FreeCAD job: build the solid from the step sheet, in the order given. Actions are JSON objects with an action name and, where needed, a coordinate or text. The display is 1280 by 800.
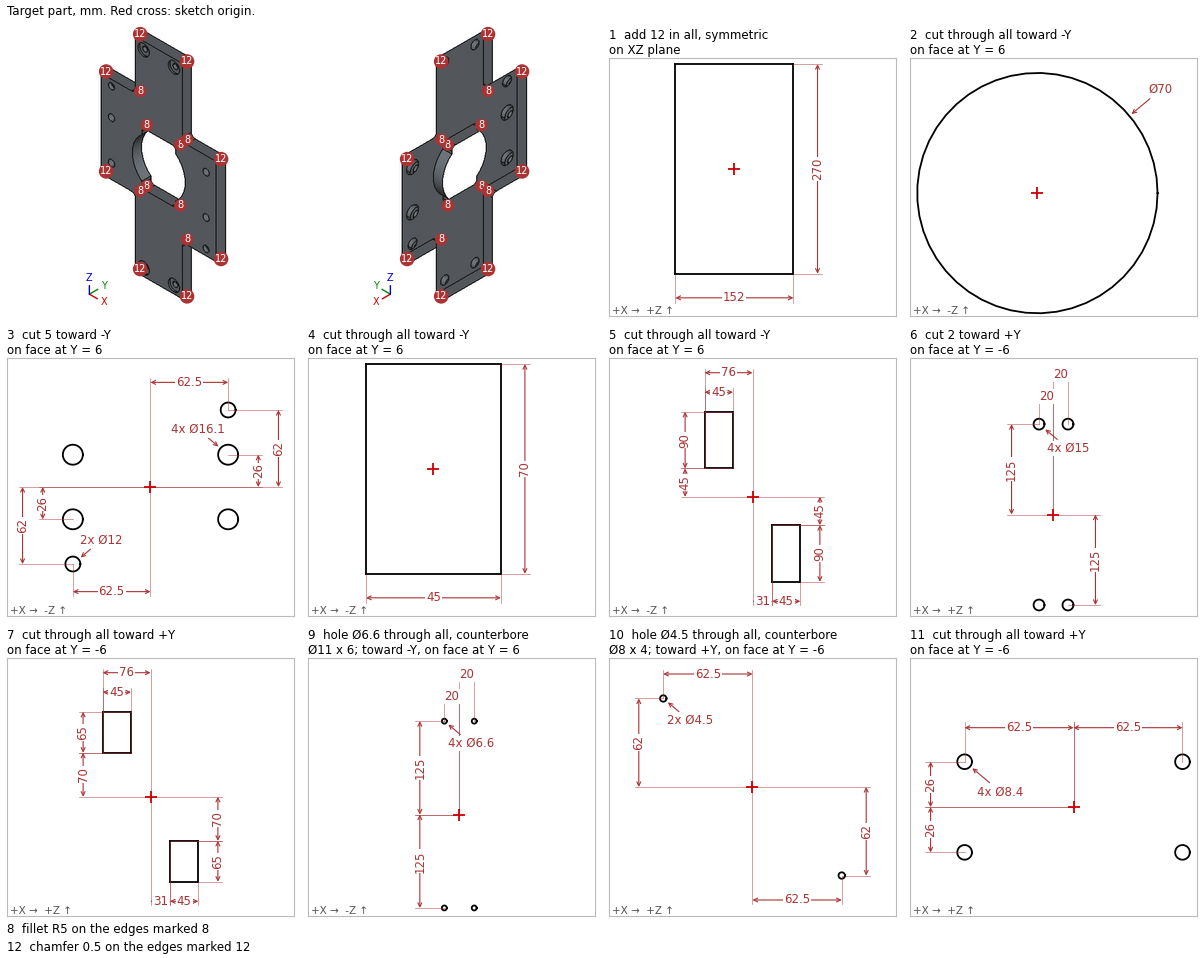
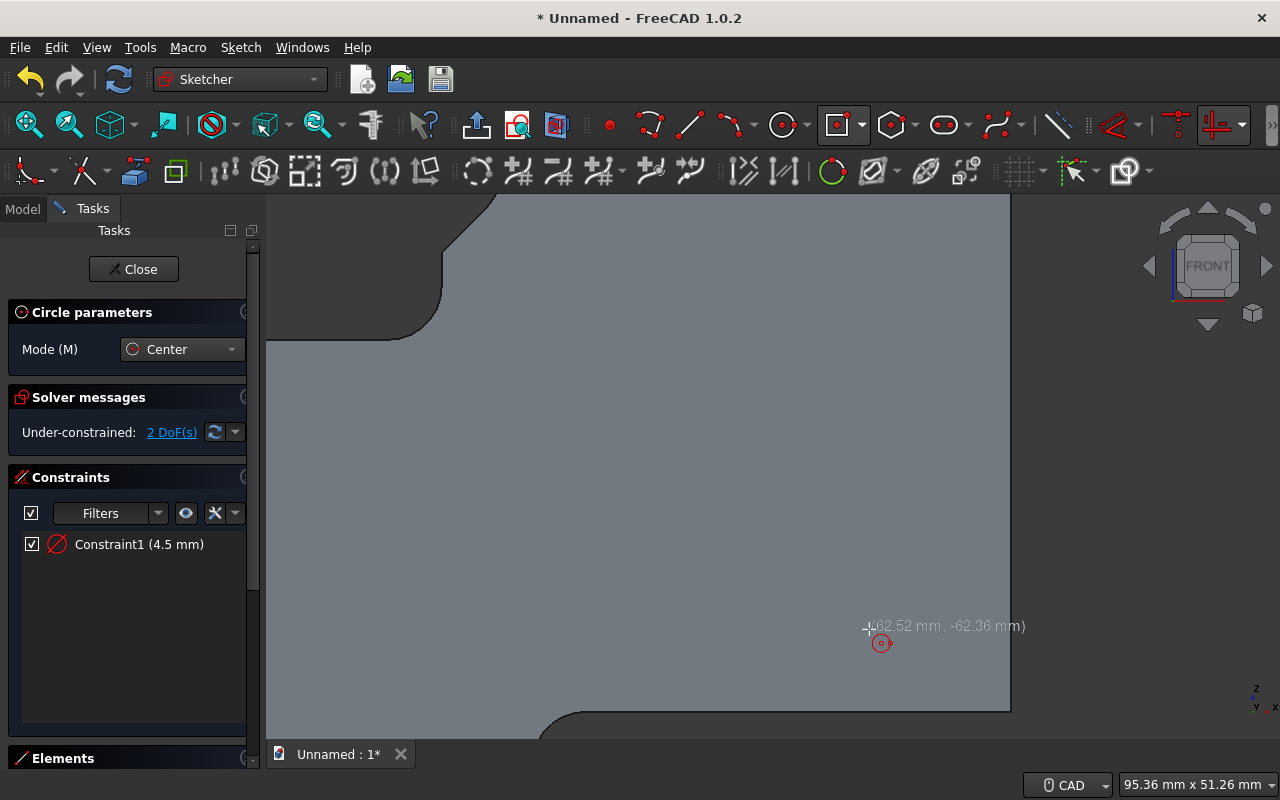
{"action": "scroll", "coordinate": [869, 630], "scroll_direction": "down", "scroll_amount": 7}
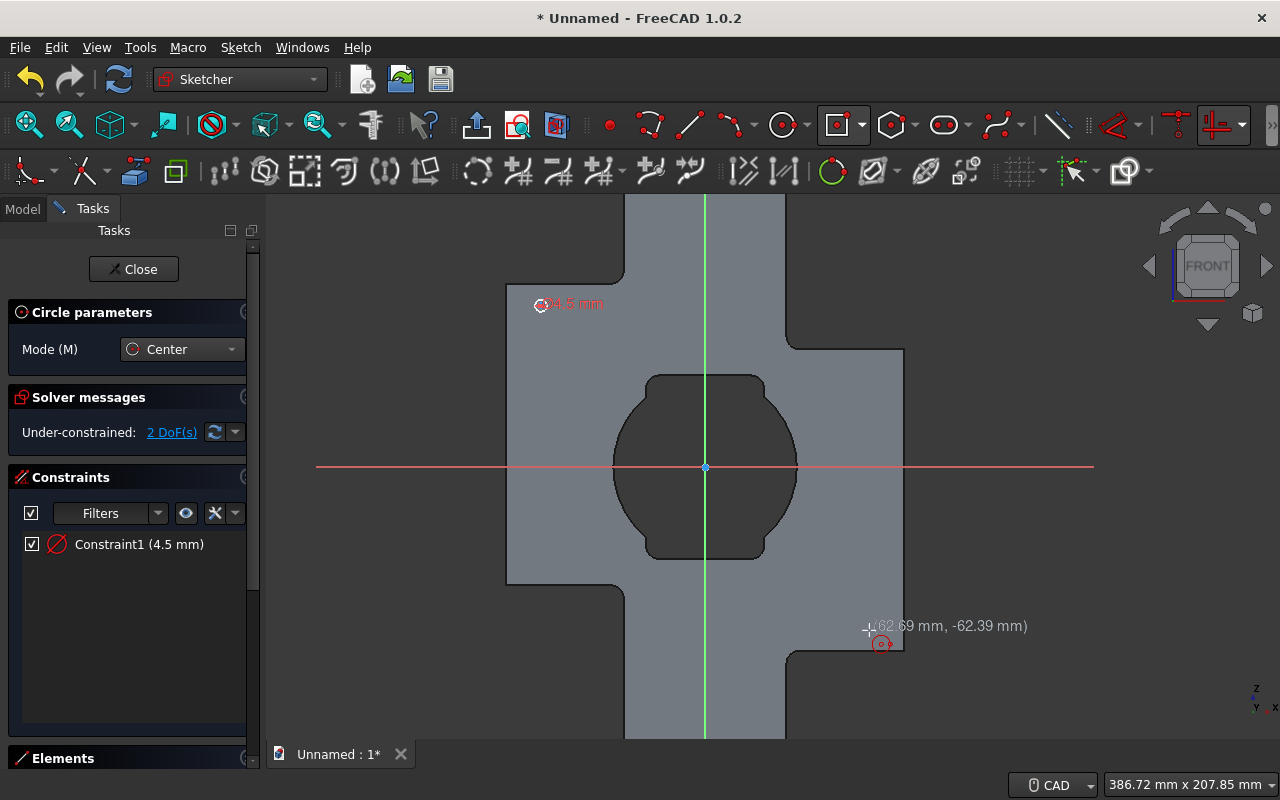
{"action": "left_click", "coordinate": [869, 630]}
{"action": "mouse_move", "coordinate": [873, 626]}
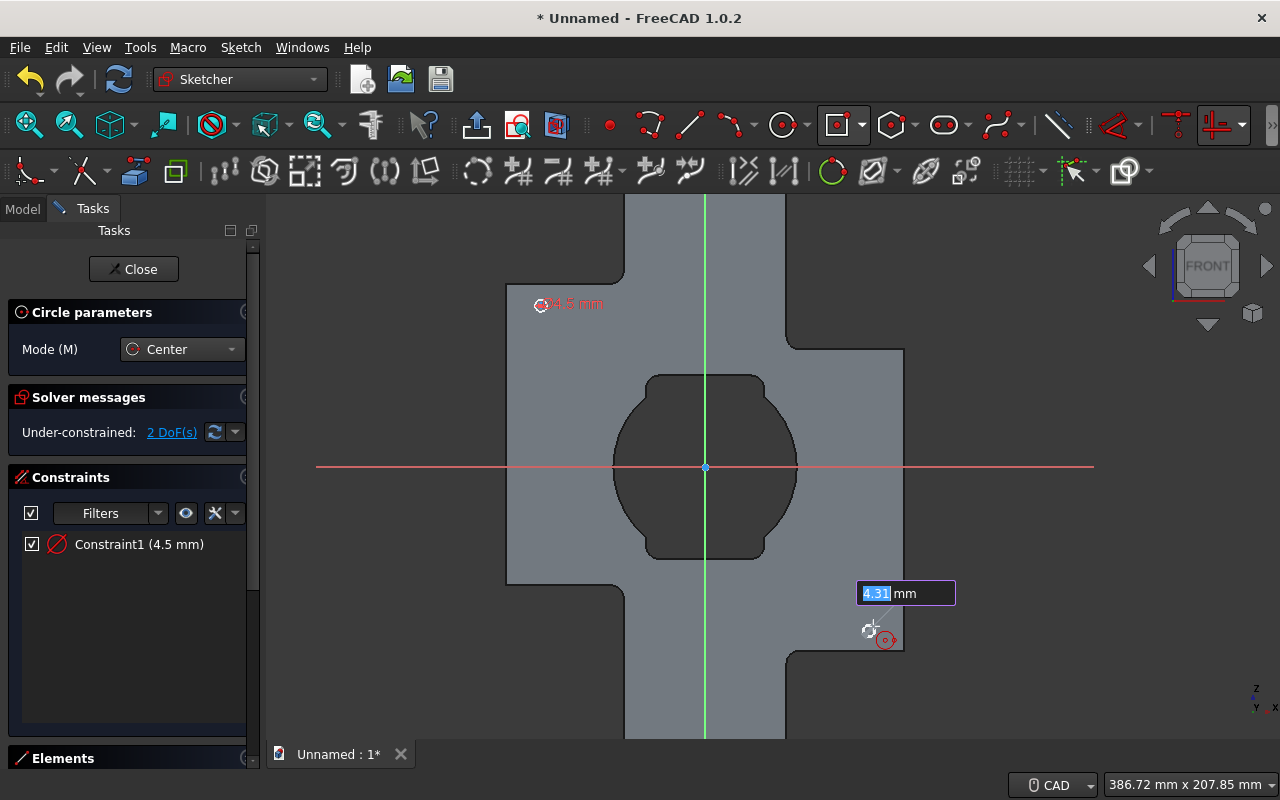
{"action": "type", "text": "4.5"}
{"action": "key", "text": "Return"}
{"action": "key", "text": "Escape"}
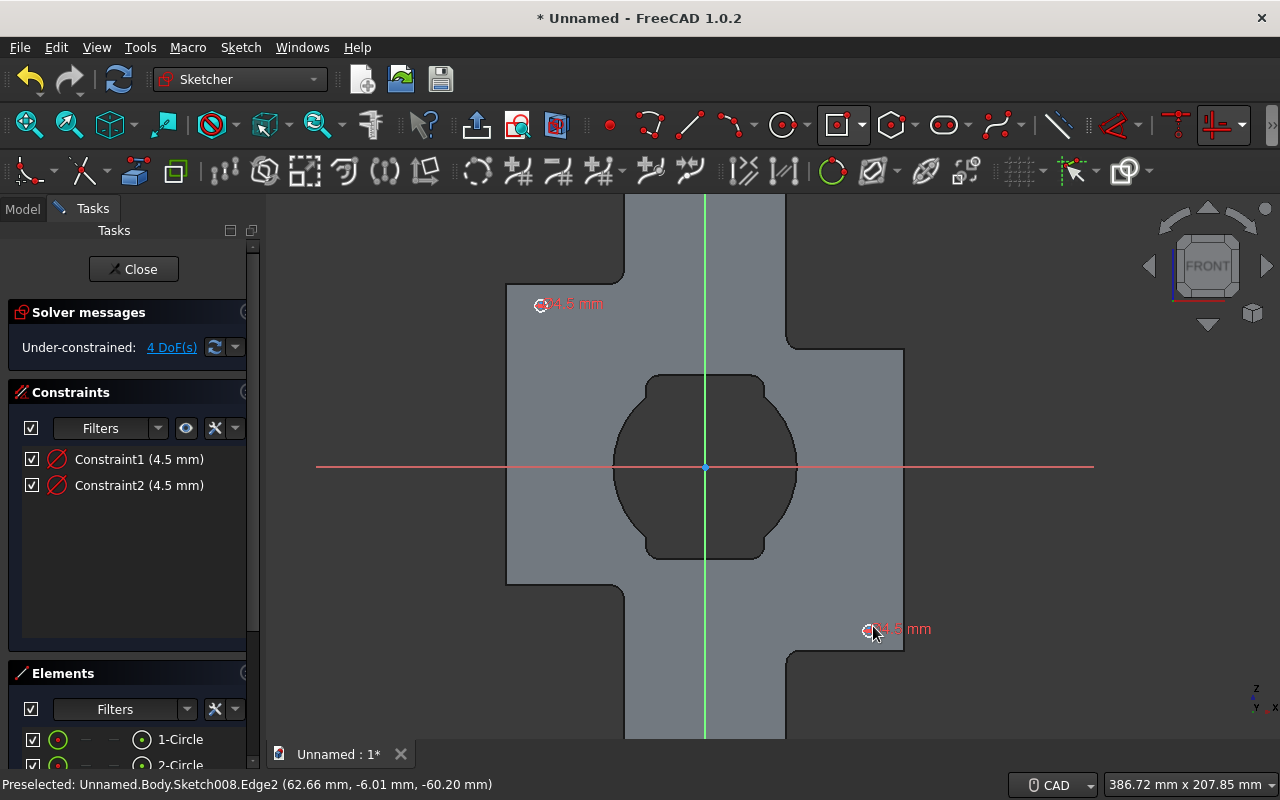
{"action": "key", "text": "d"}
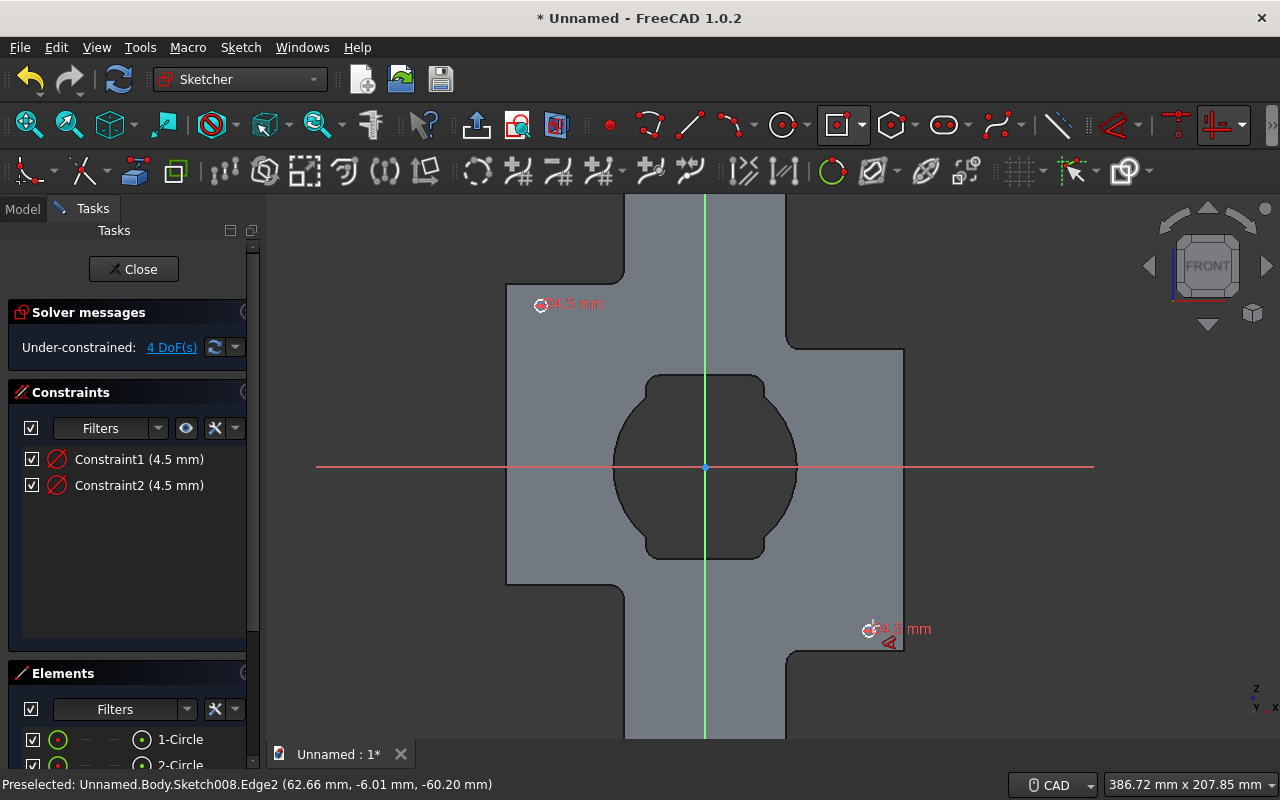
{"action": "left_click", "coordinate": [541, 306]}
{"action": "left_click", "coordinate": [507, 387]}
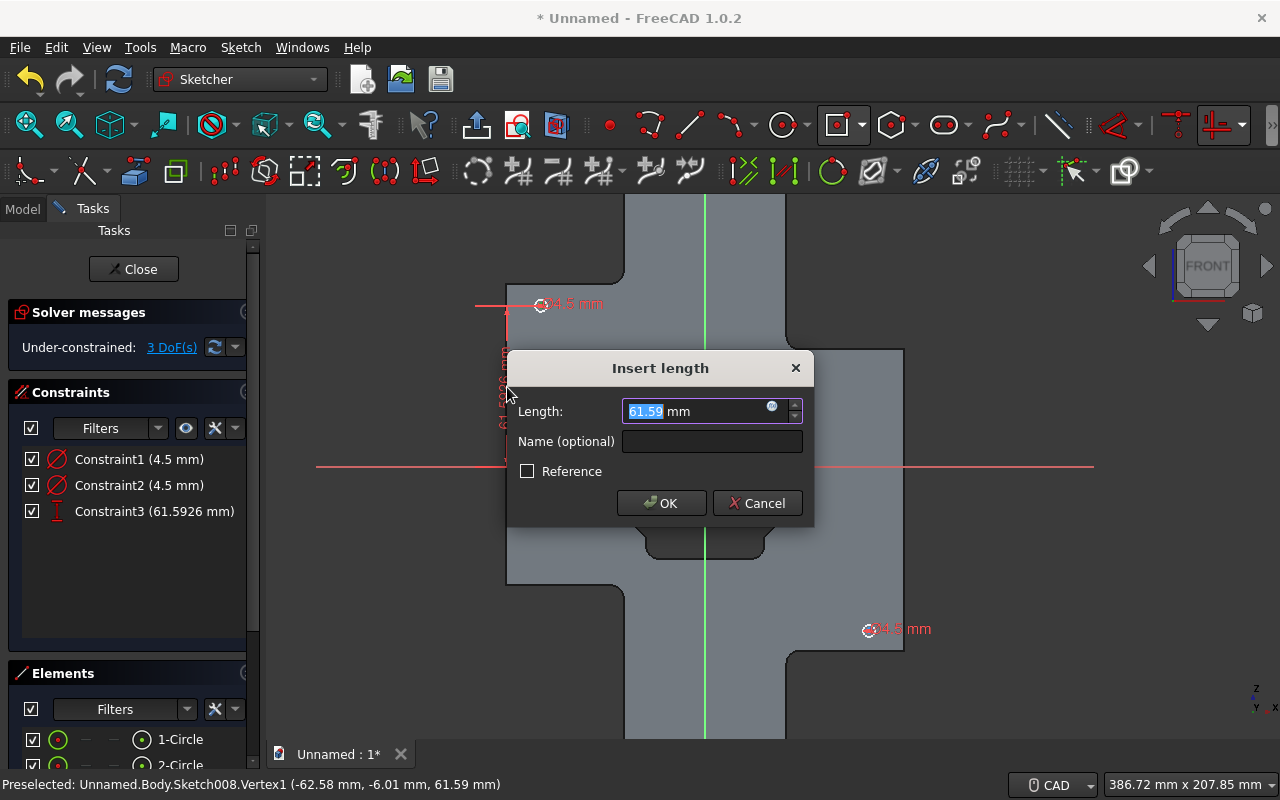
{"action": "type", "text": "62"}
{"action": "key", "text": "Return"}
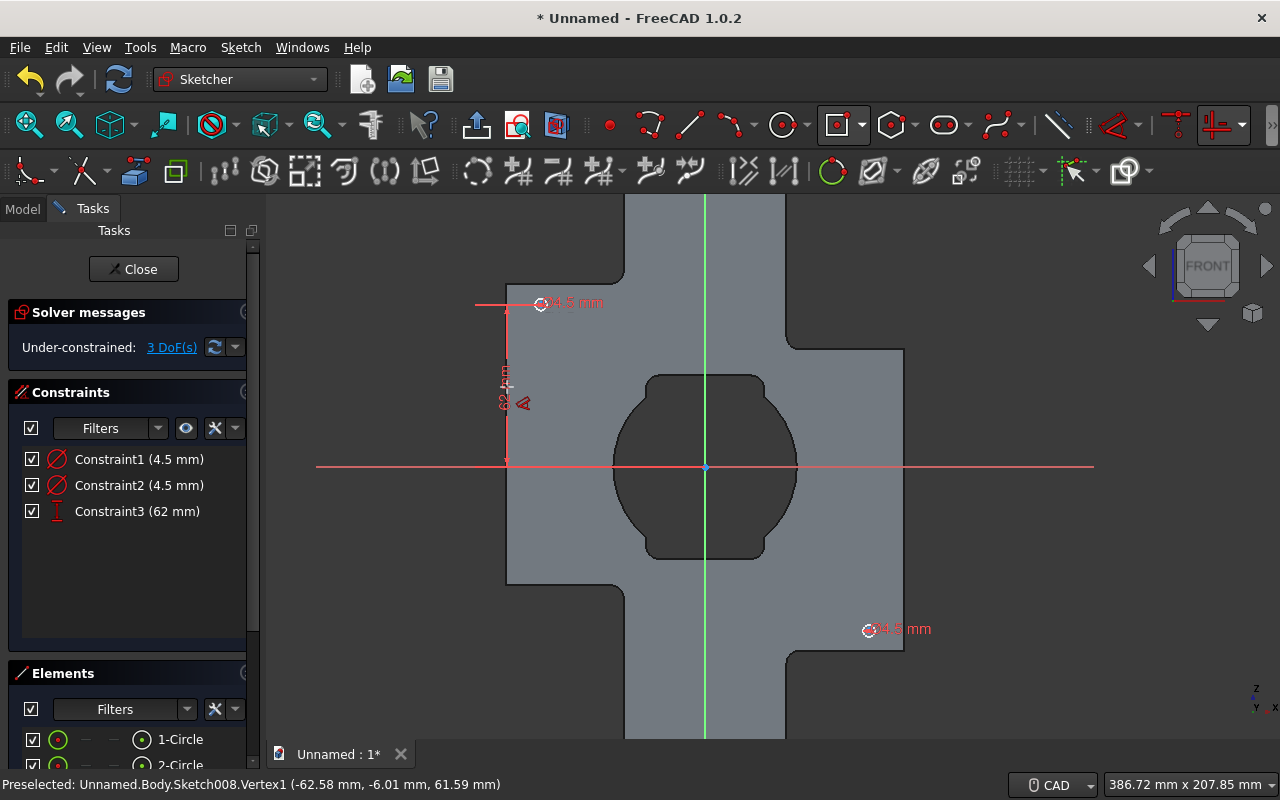
{"action": "left_click", "coordinate": [869, 631]}
{"action": "left_click", "coordinate": [903, 549]}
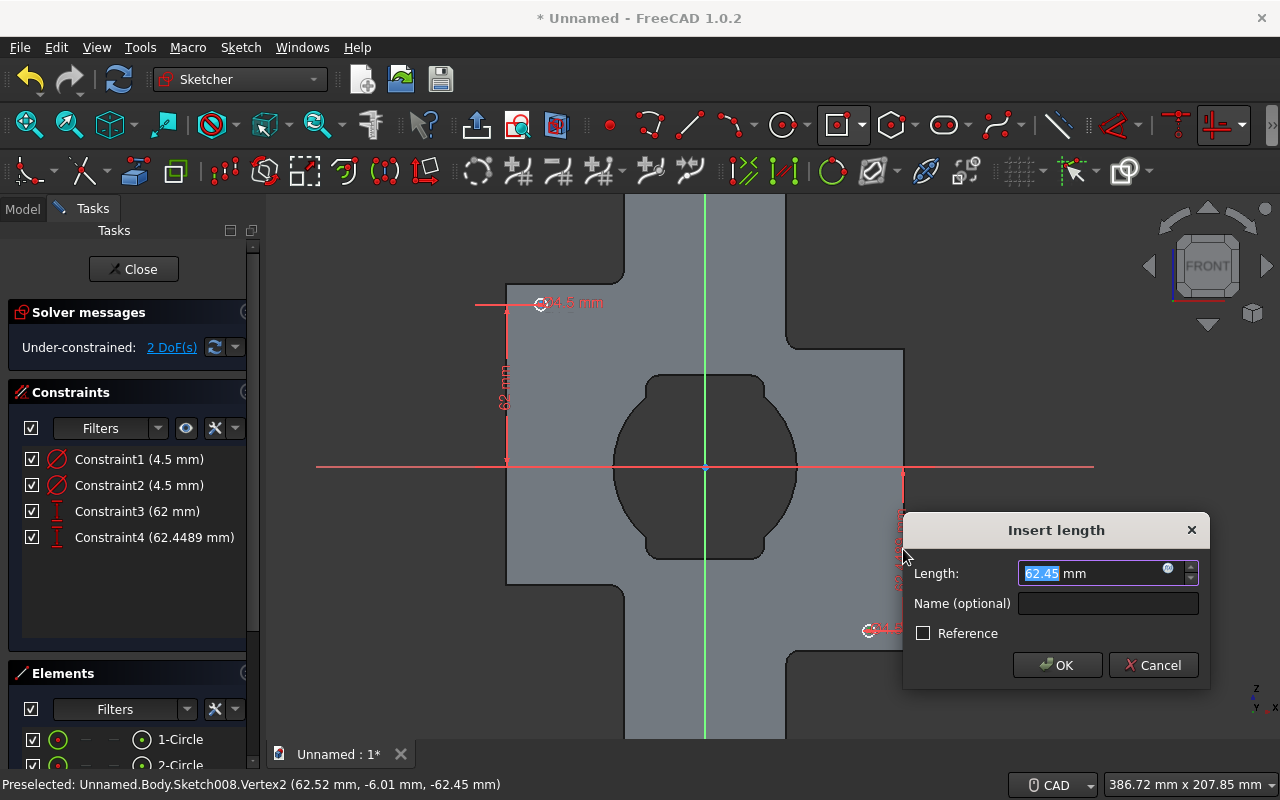
{"action": "type", "text": "62"}
{"action": "key", "text": "Return"}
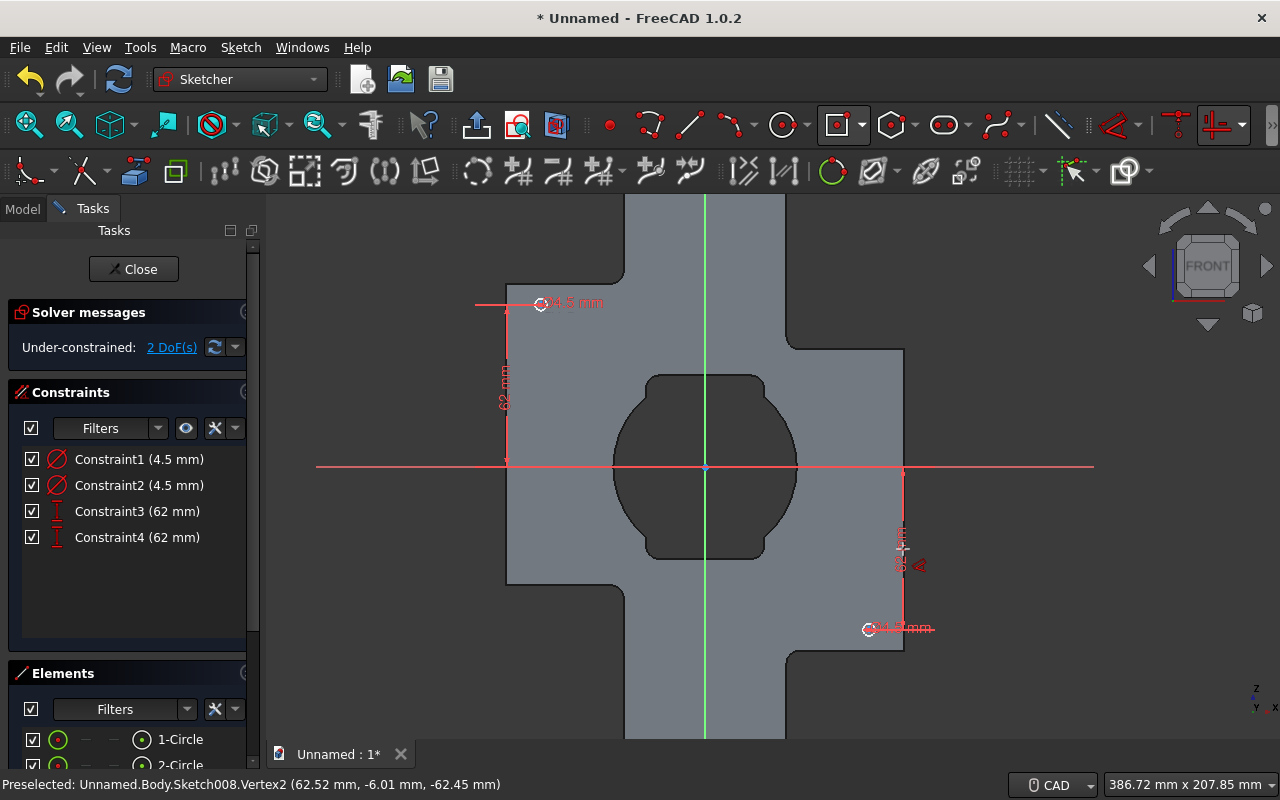
{"action": "left_click", "coordinate": [541, 305]}
{"action": "left_click", "coordinate": [623, 271]}